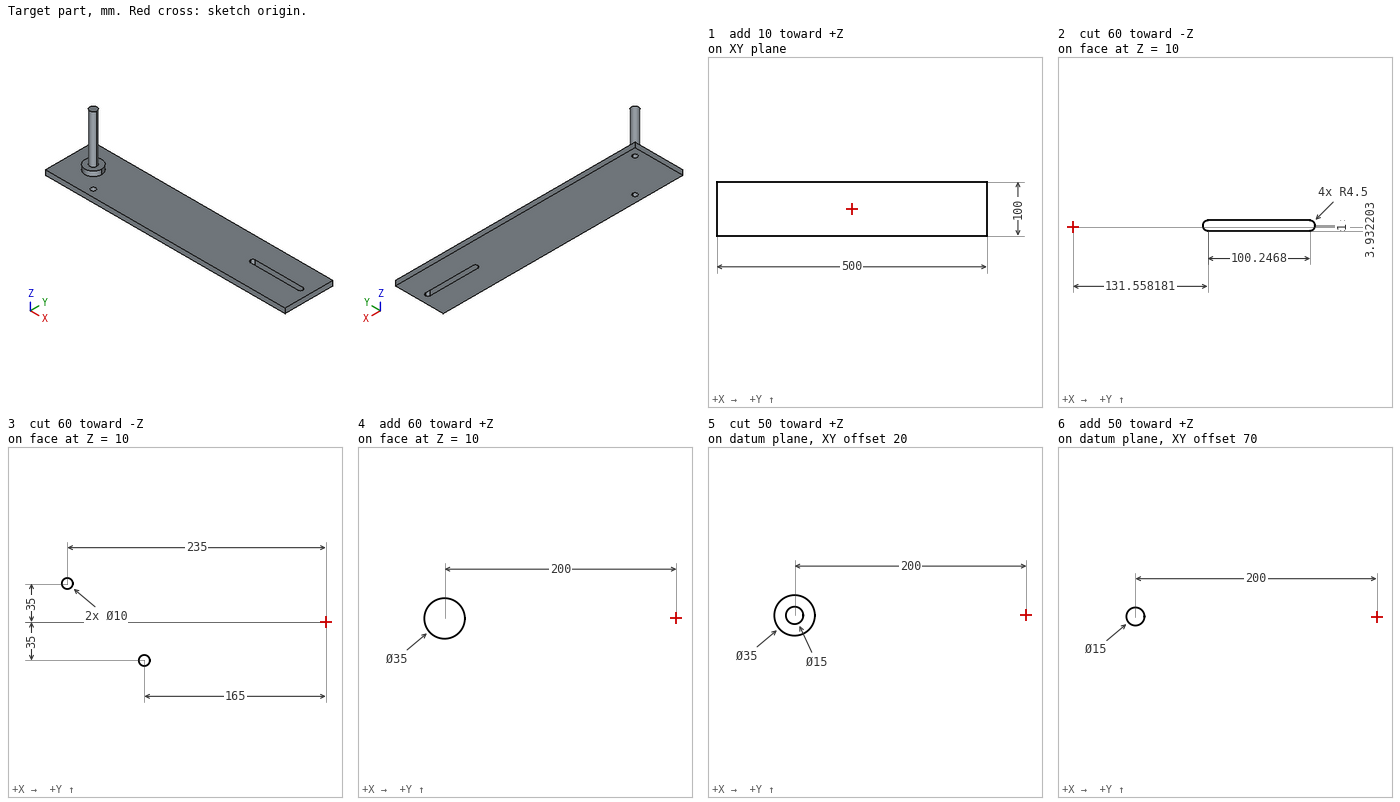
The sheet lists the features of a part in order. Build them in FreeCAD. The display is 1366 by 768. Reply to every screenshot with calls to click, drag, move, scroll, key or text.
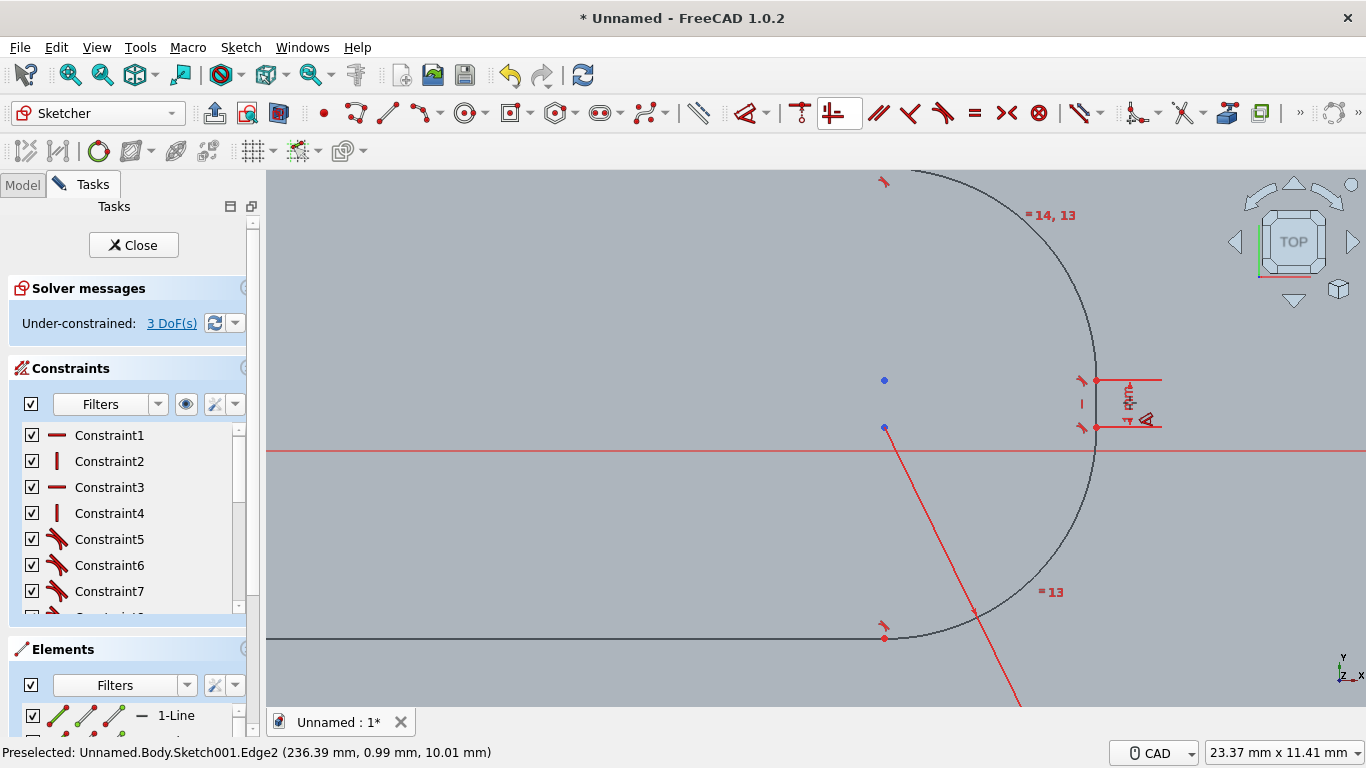
scroll(1085, 441, down, 14)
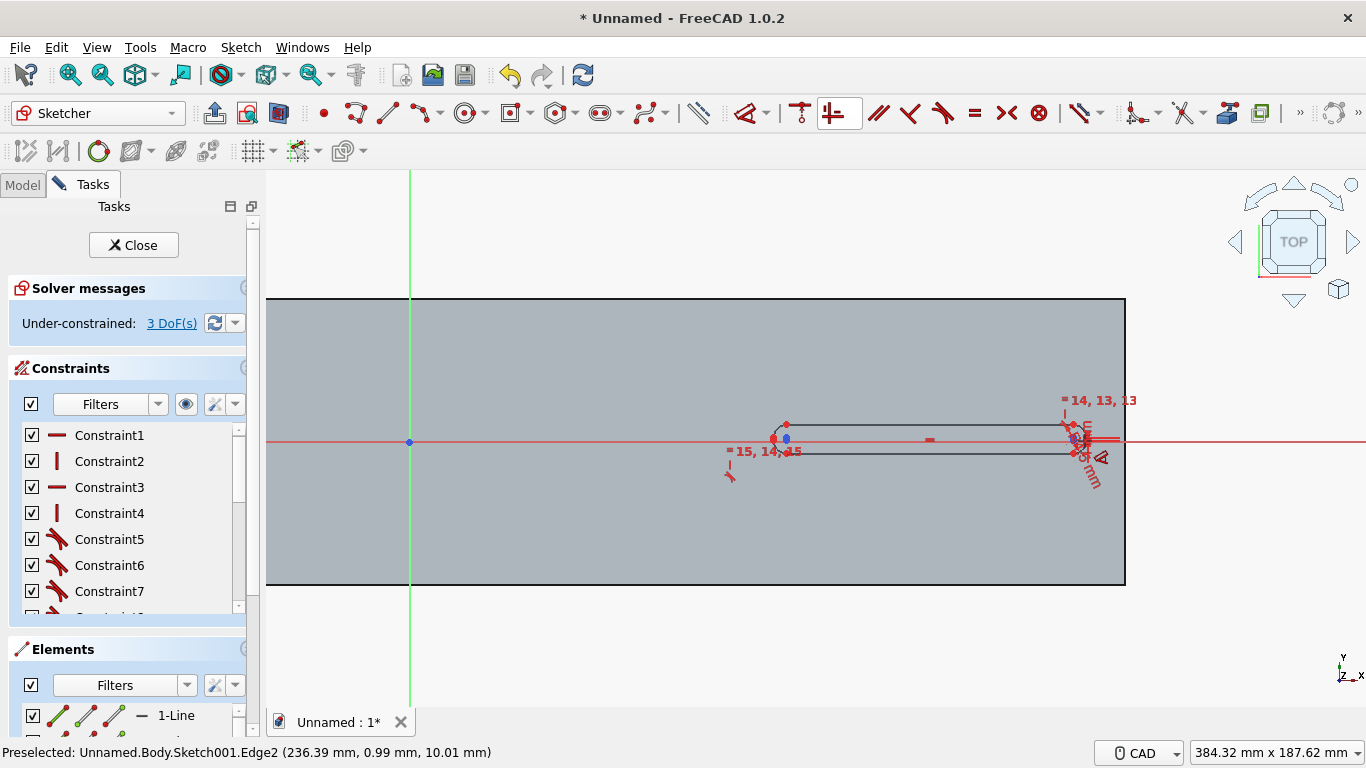
click(873, 454)
click(930, 488)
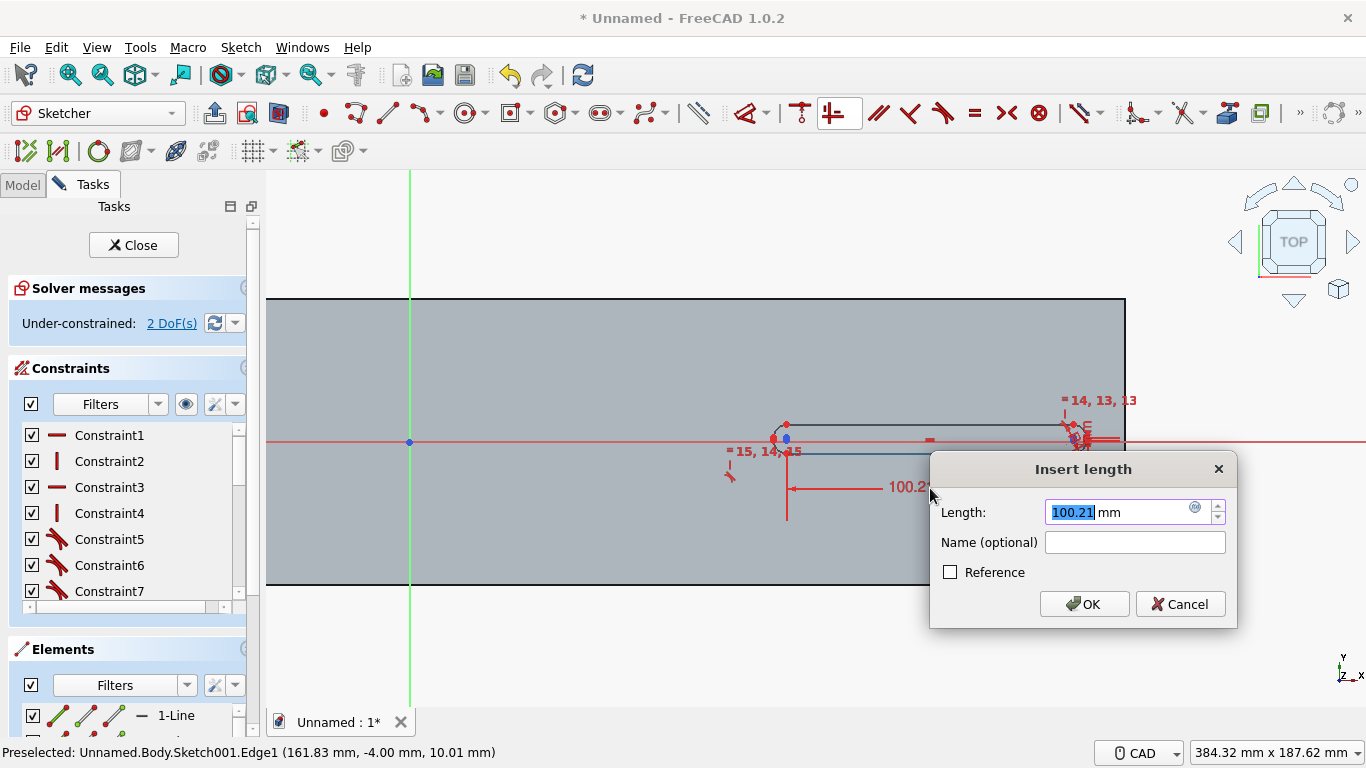
text(100.2468)
key(Return)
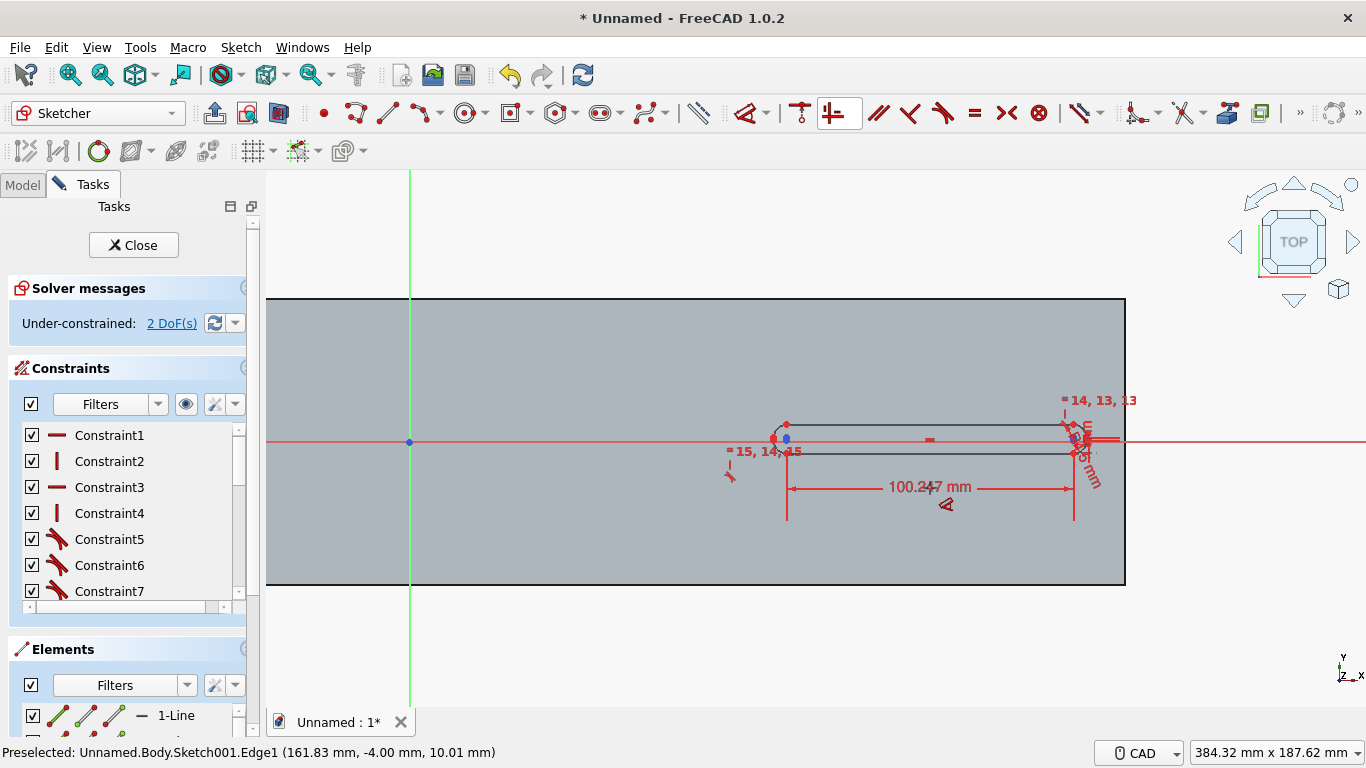
scroll(787, 454, up, 7)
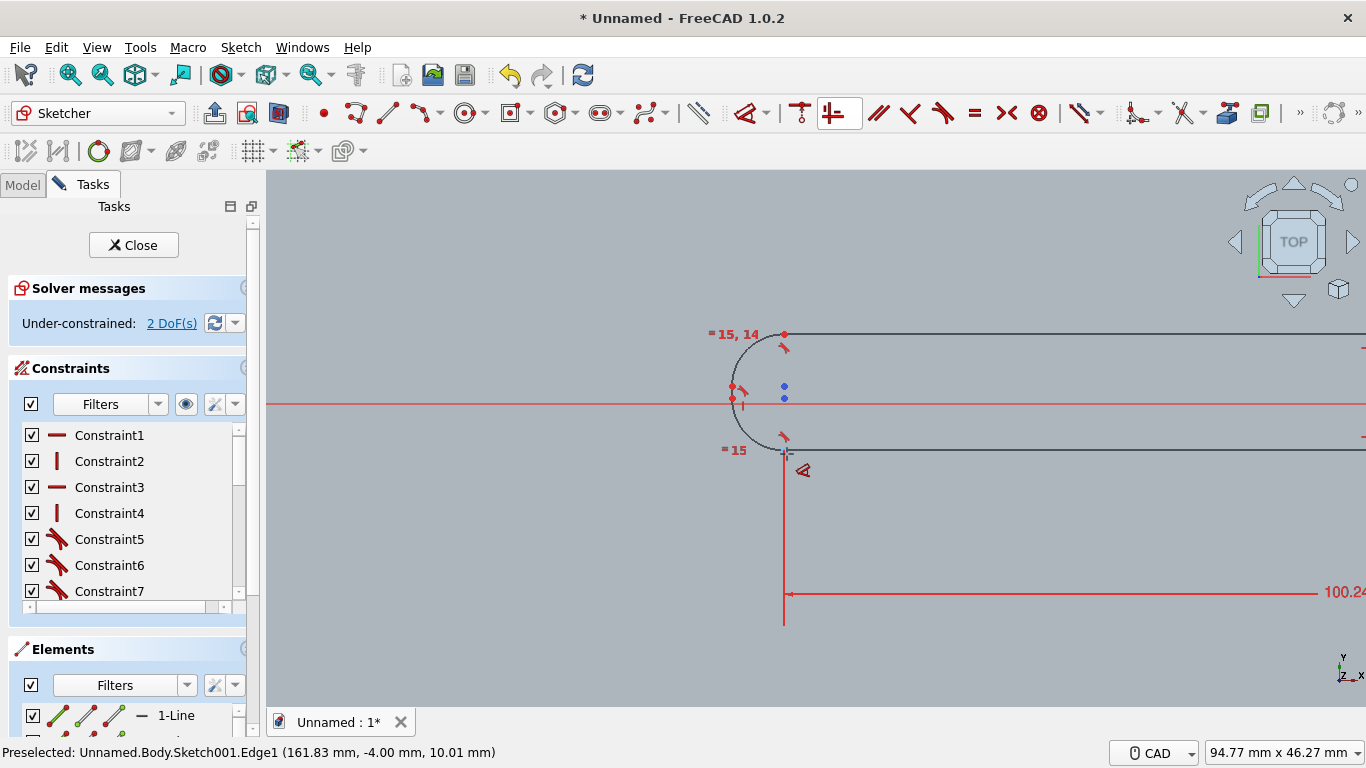
click(784, 450)
click(818, 427)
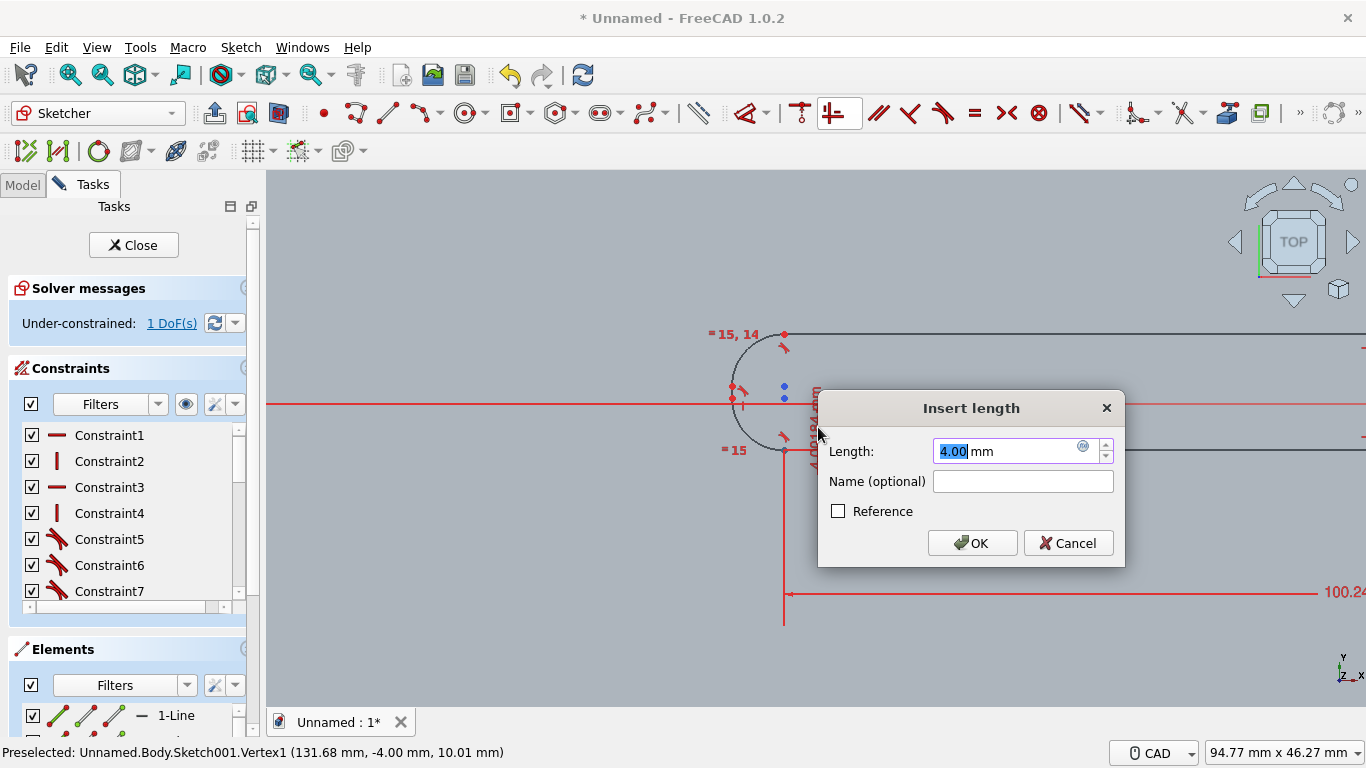
text(3.932203)
key(Return)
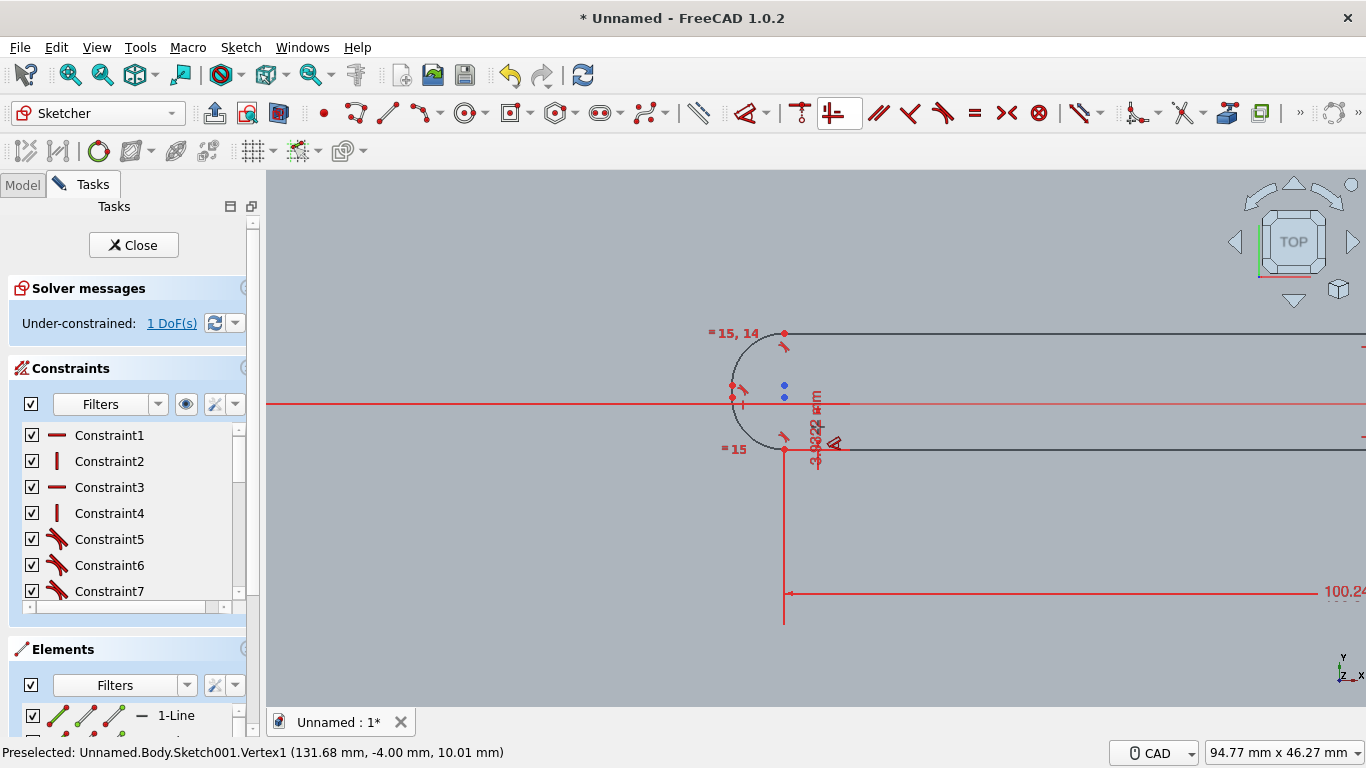
scroll(787, 454, down, 7)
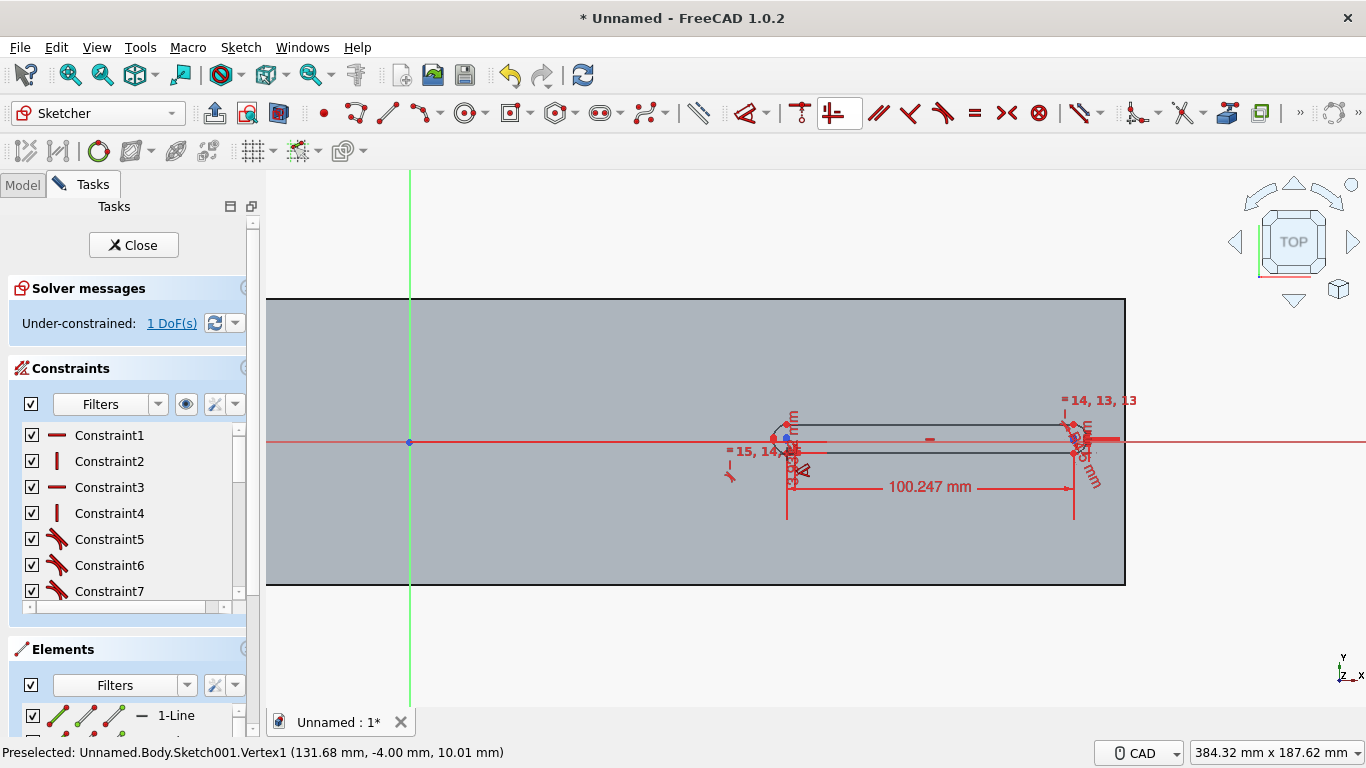
click(787, 453)
click(598, 487)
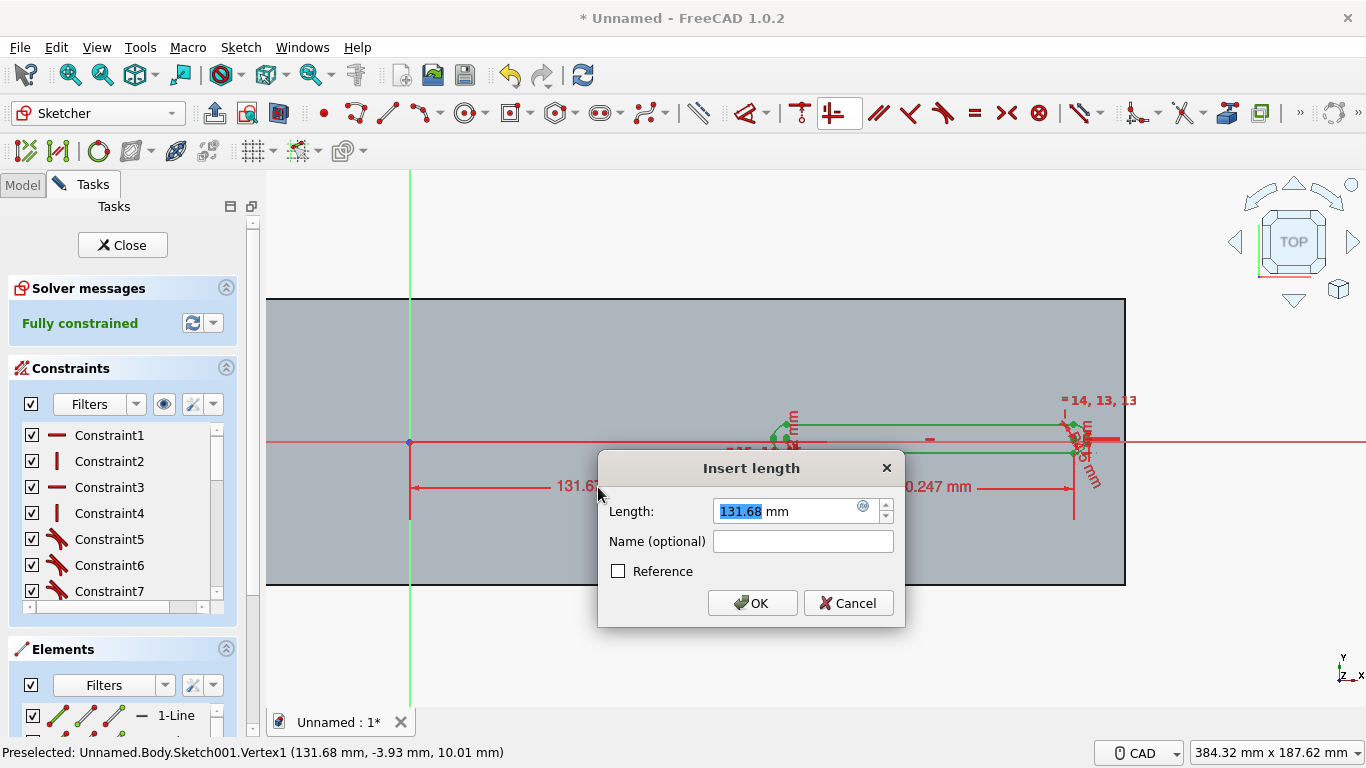
text(131.558181)
key(Return)
key(Escape)